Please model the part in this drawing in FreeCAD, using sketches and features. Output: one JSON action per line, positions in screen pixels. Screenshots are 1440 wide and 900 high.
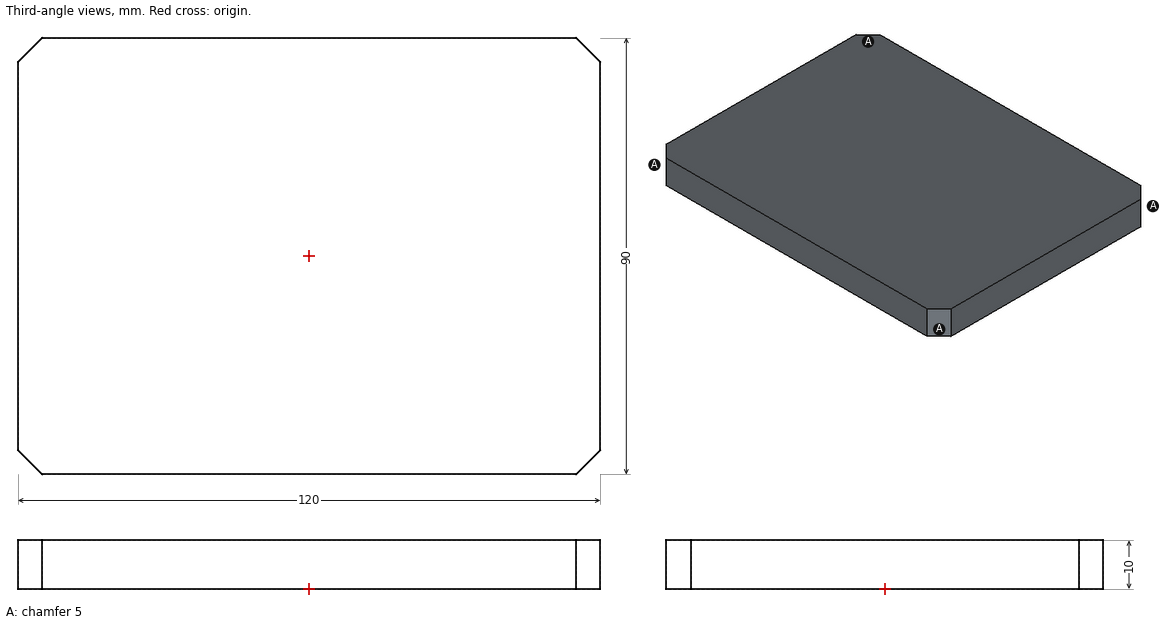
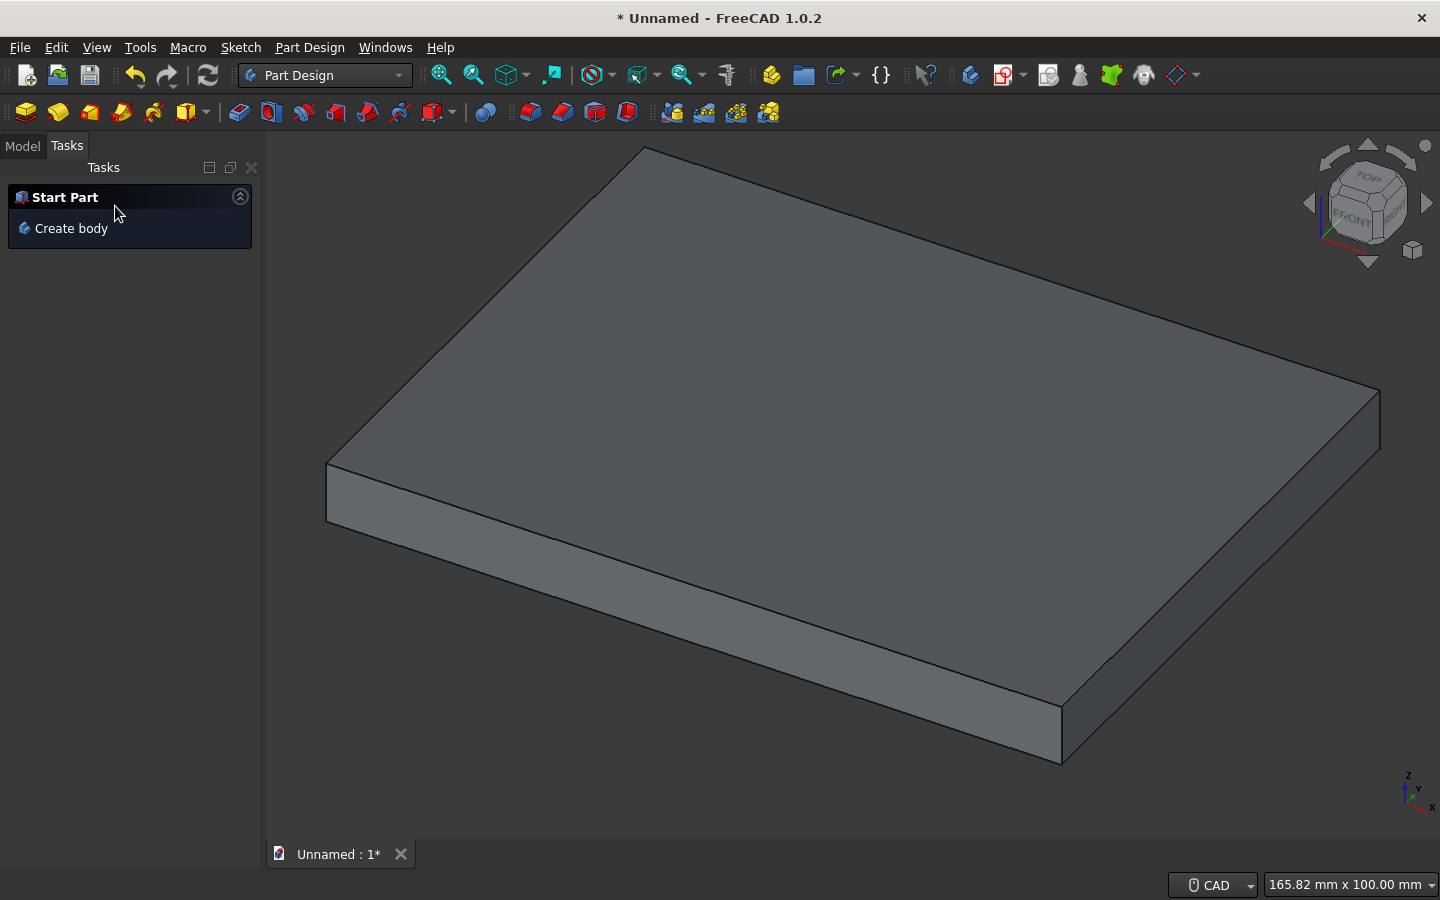
{"action": "left_click", "coordinate": [1062, 735]}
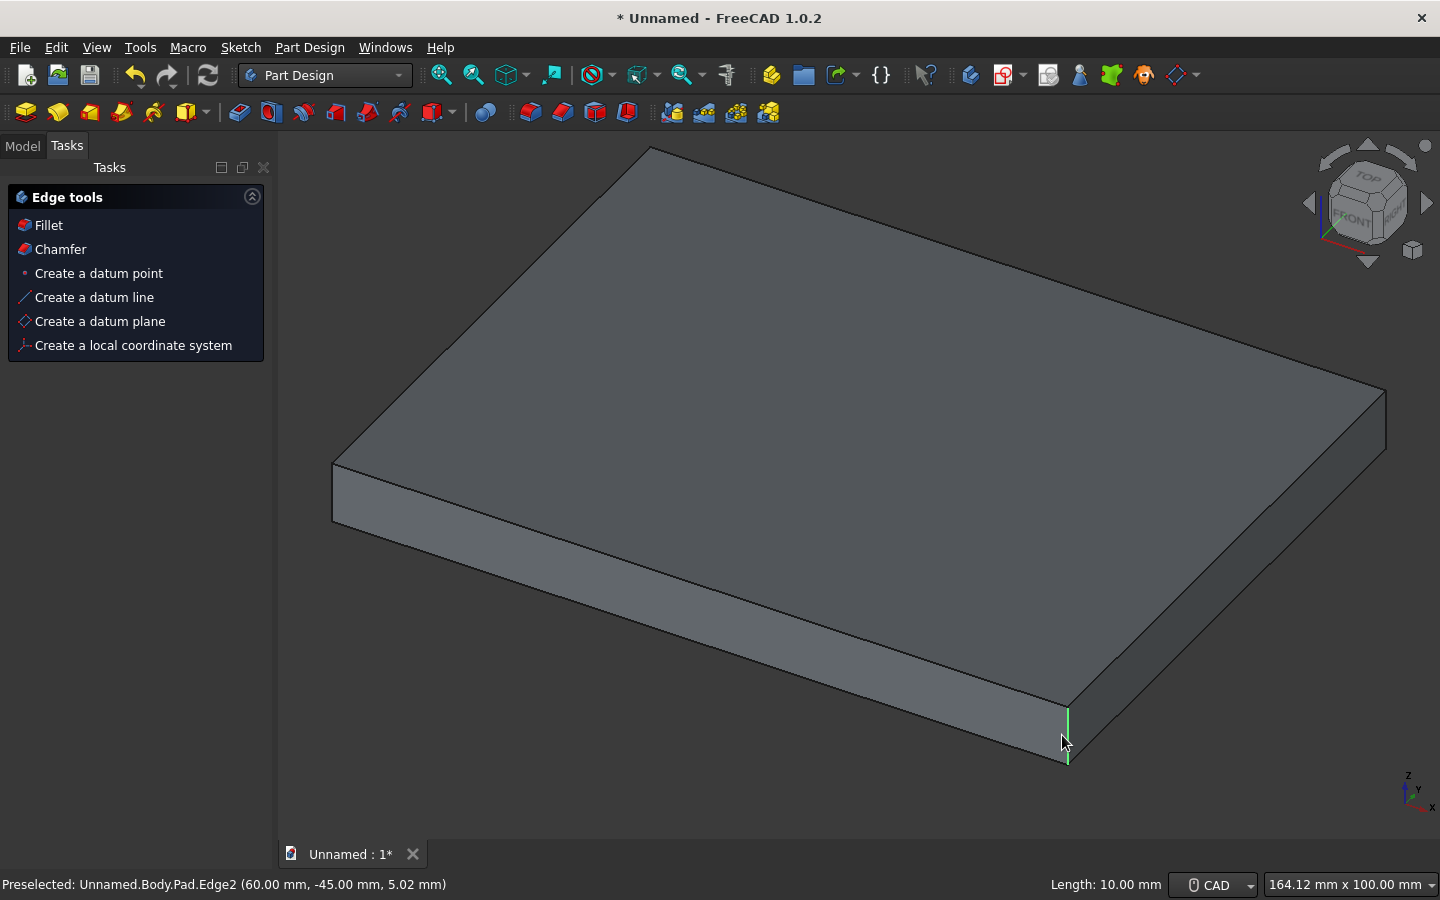
{"action": "key", "text": "0"}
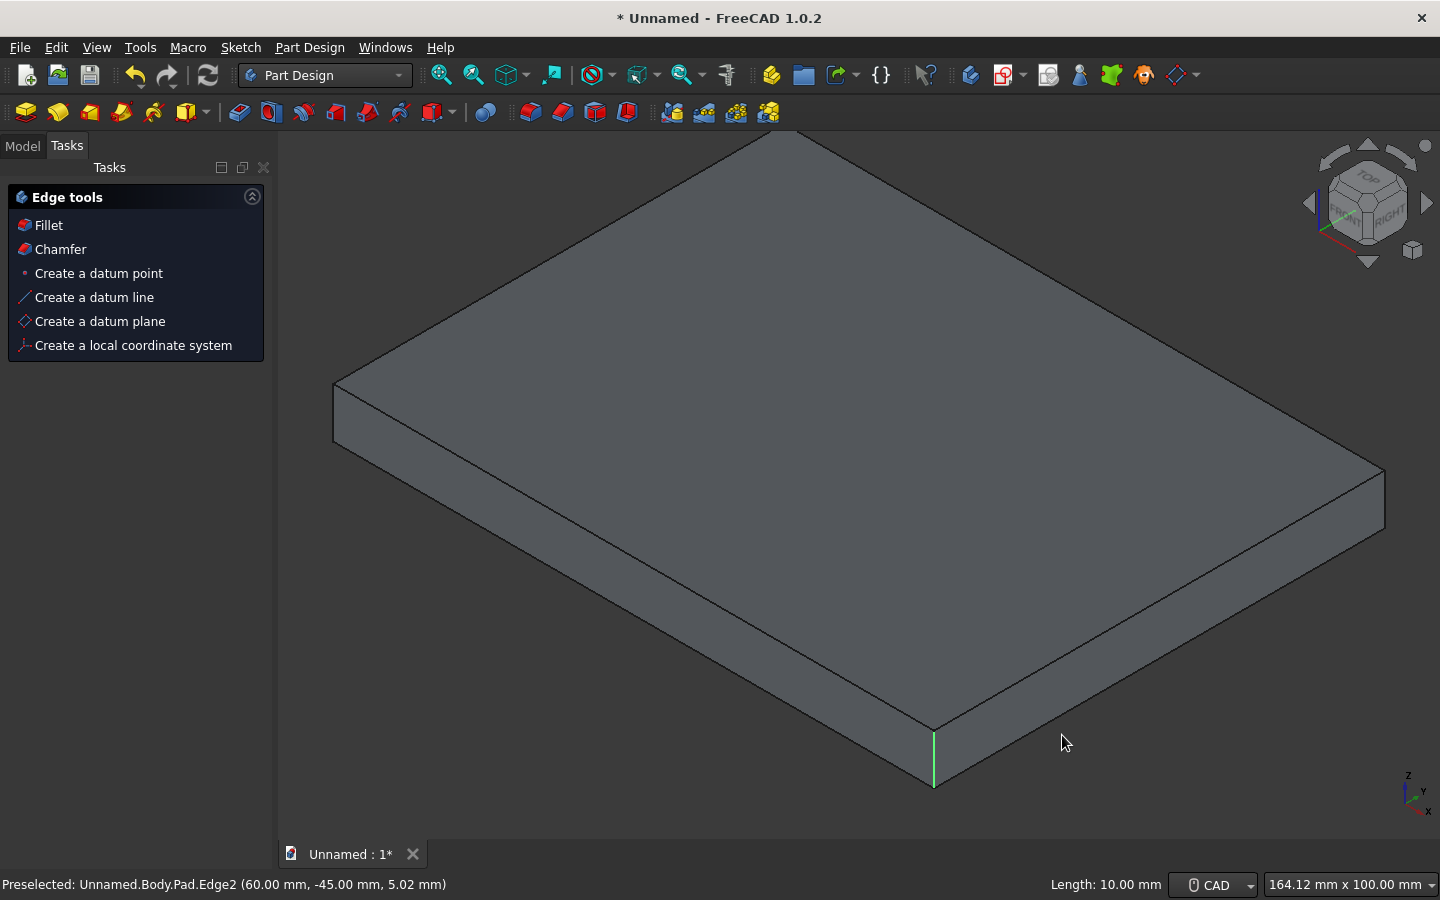
{"action": "left_click", "coordinate": [442, 76]}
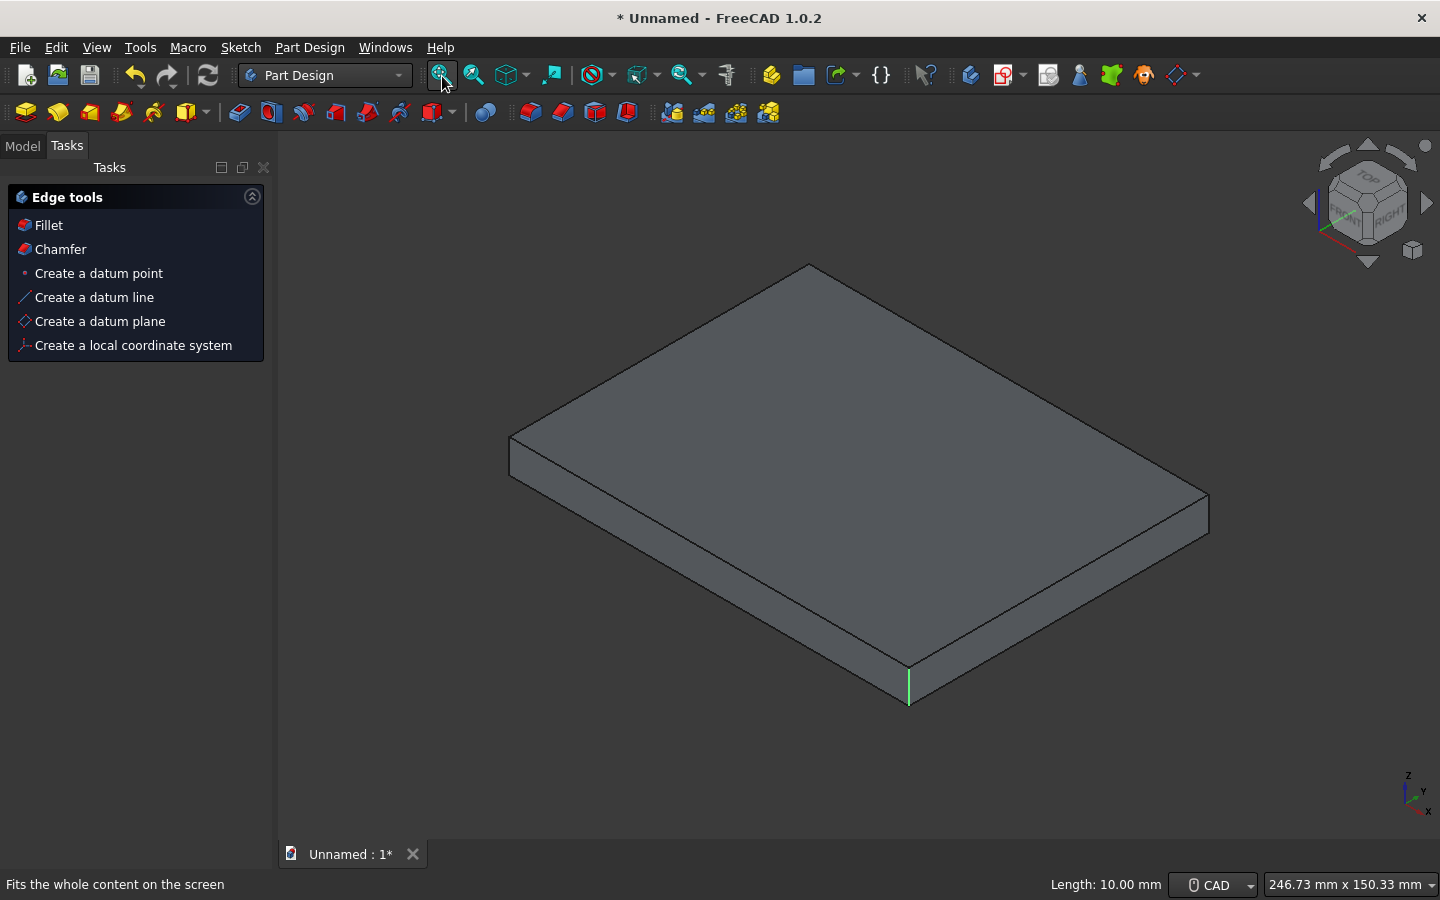
{"action": "key", "text": "2"}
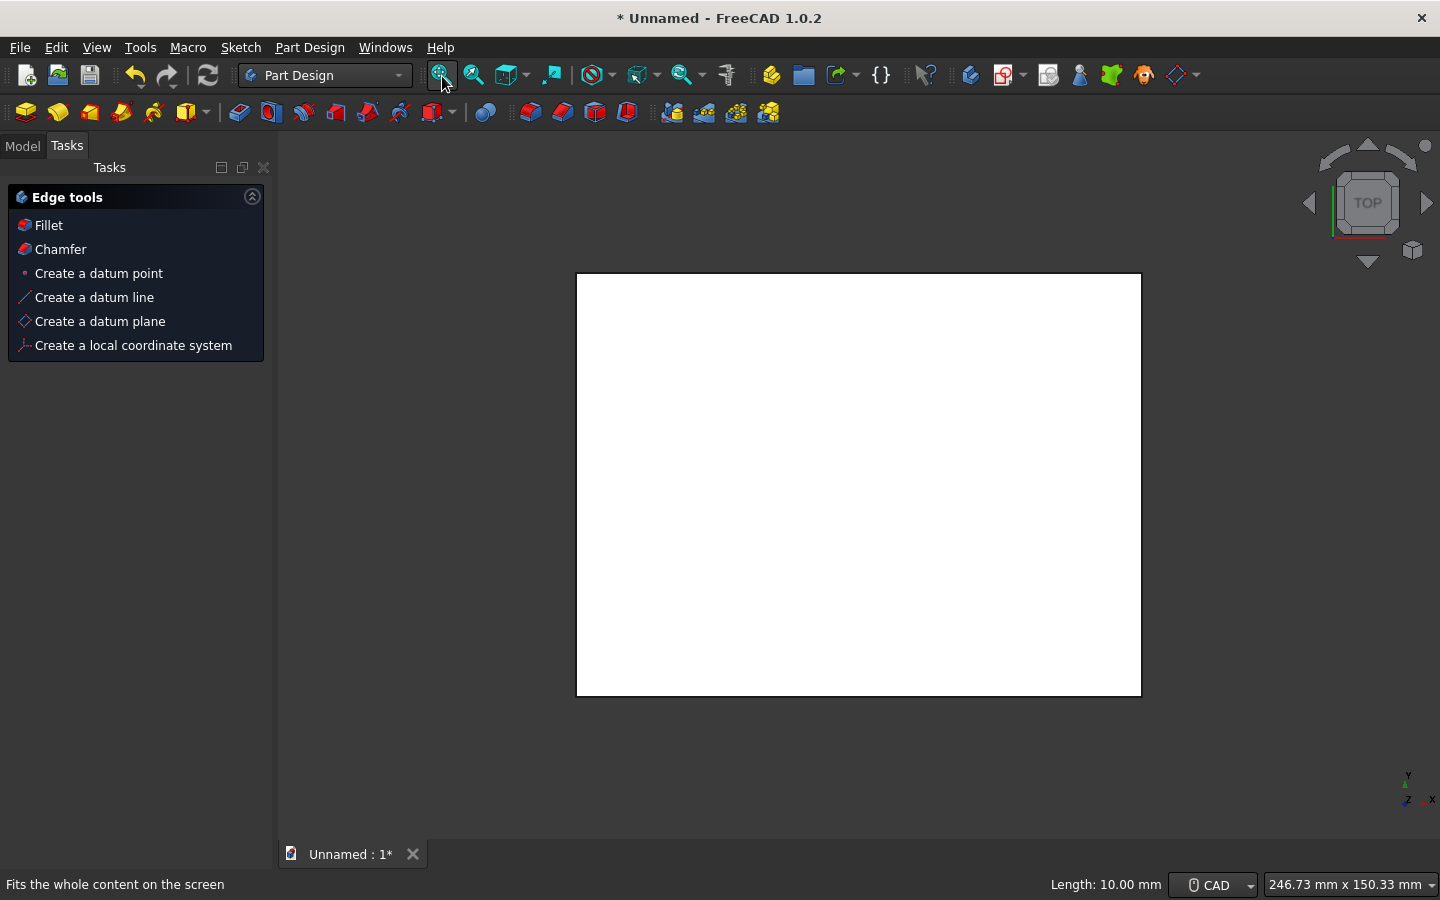
{"action": "key", "text": "1"}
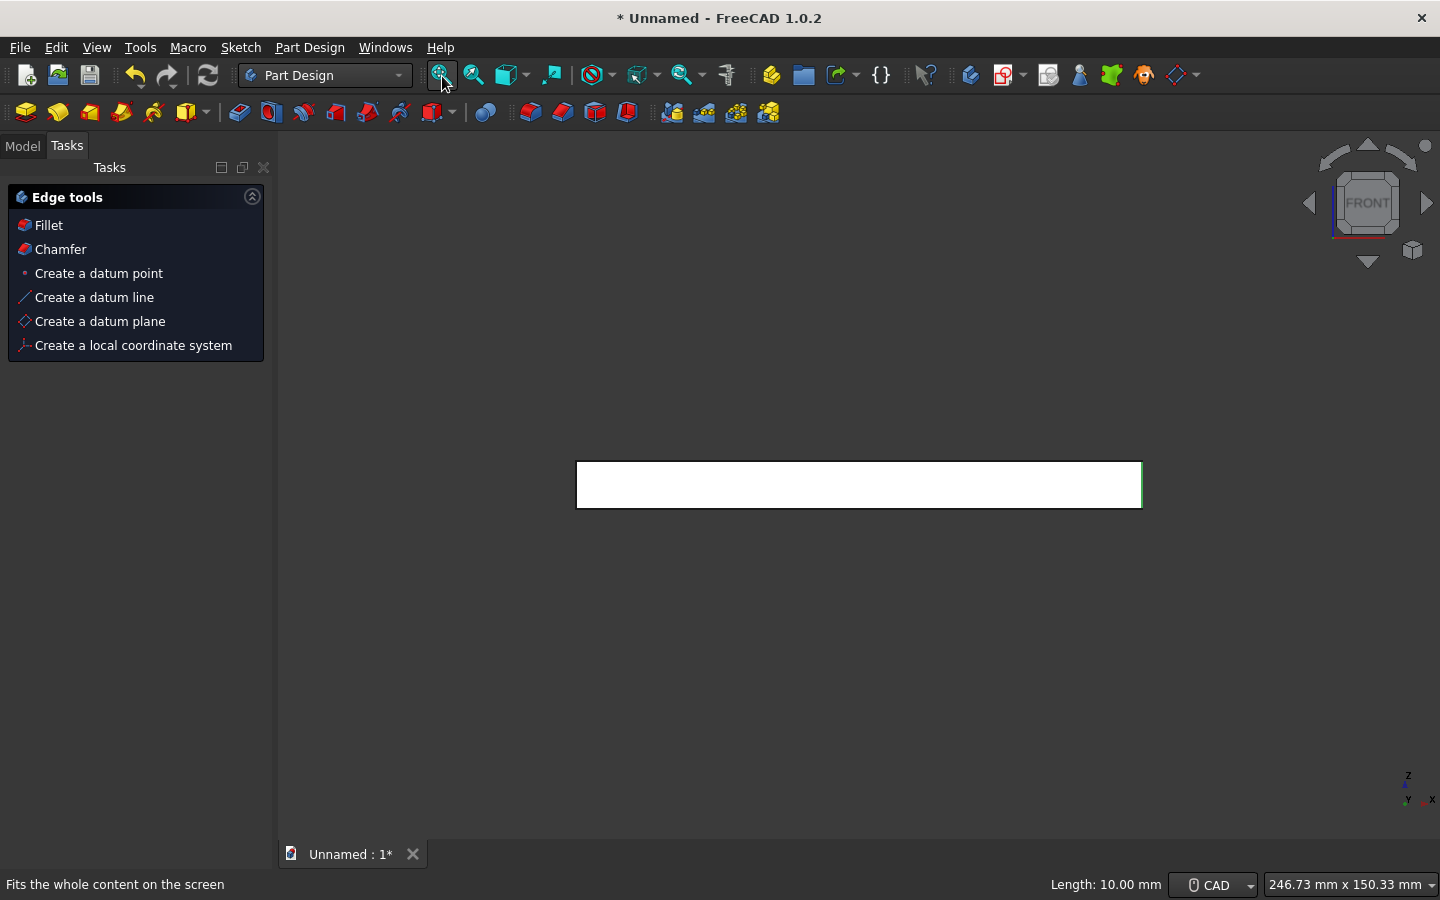
{"action": "left_click", "coordinate": [576, 484], "text": "ctrl"}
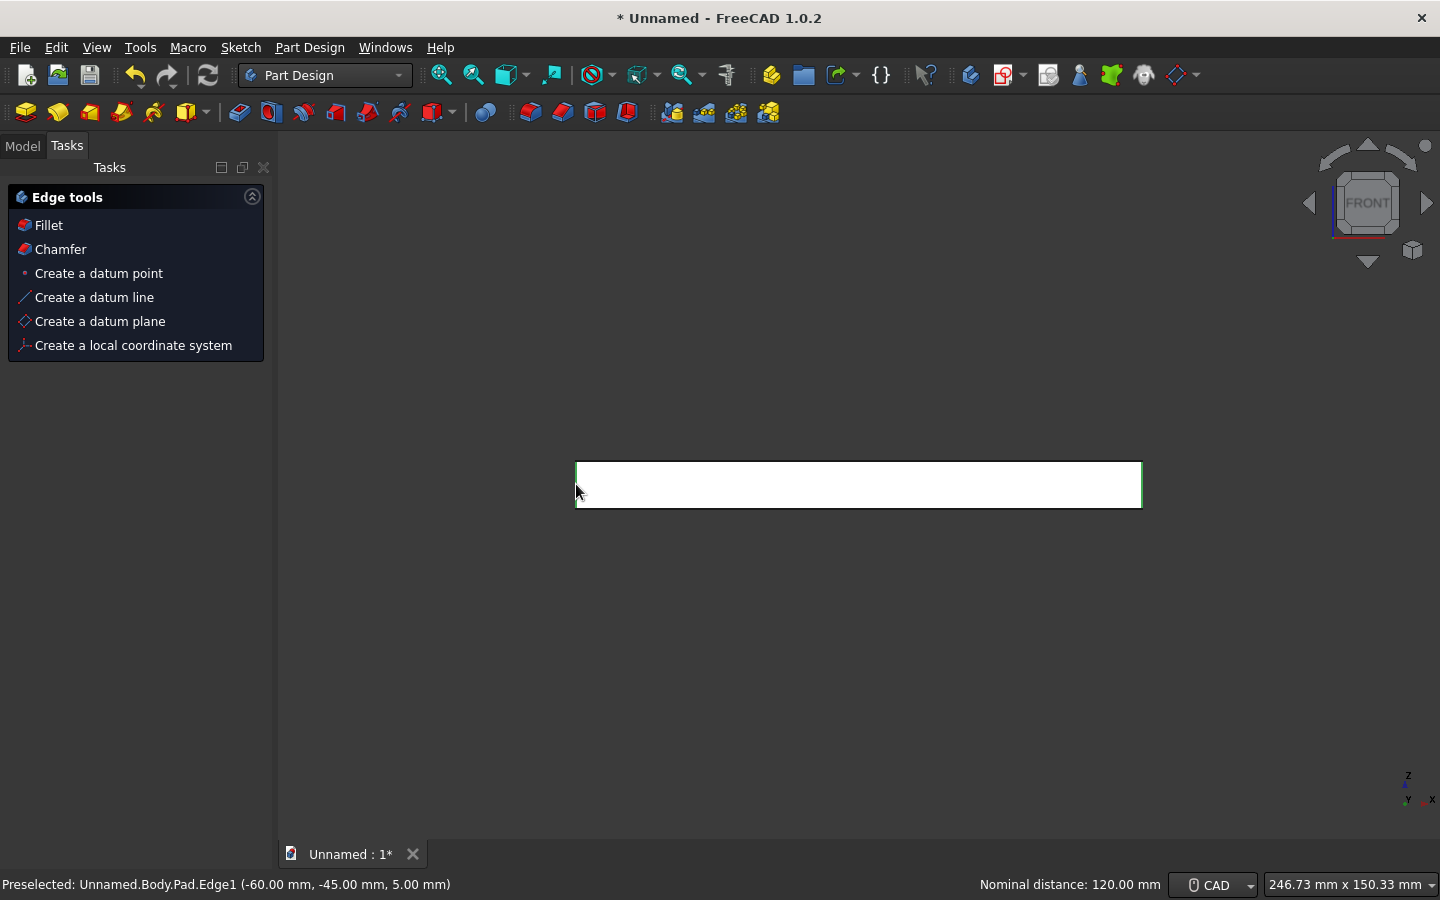
{"action": "key", "text": "3"}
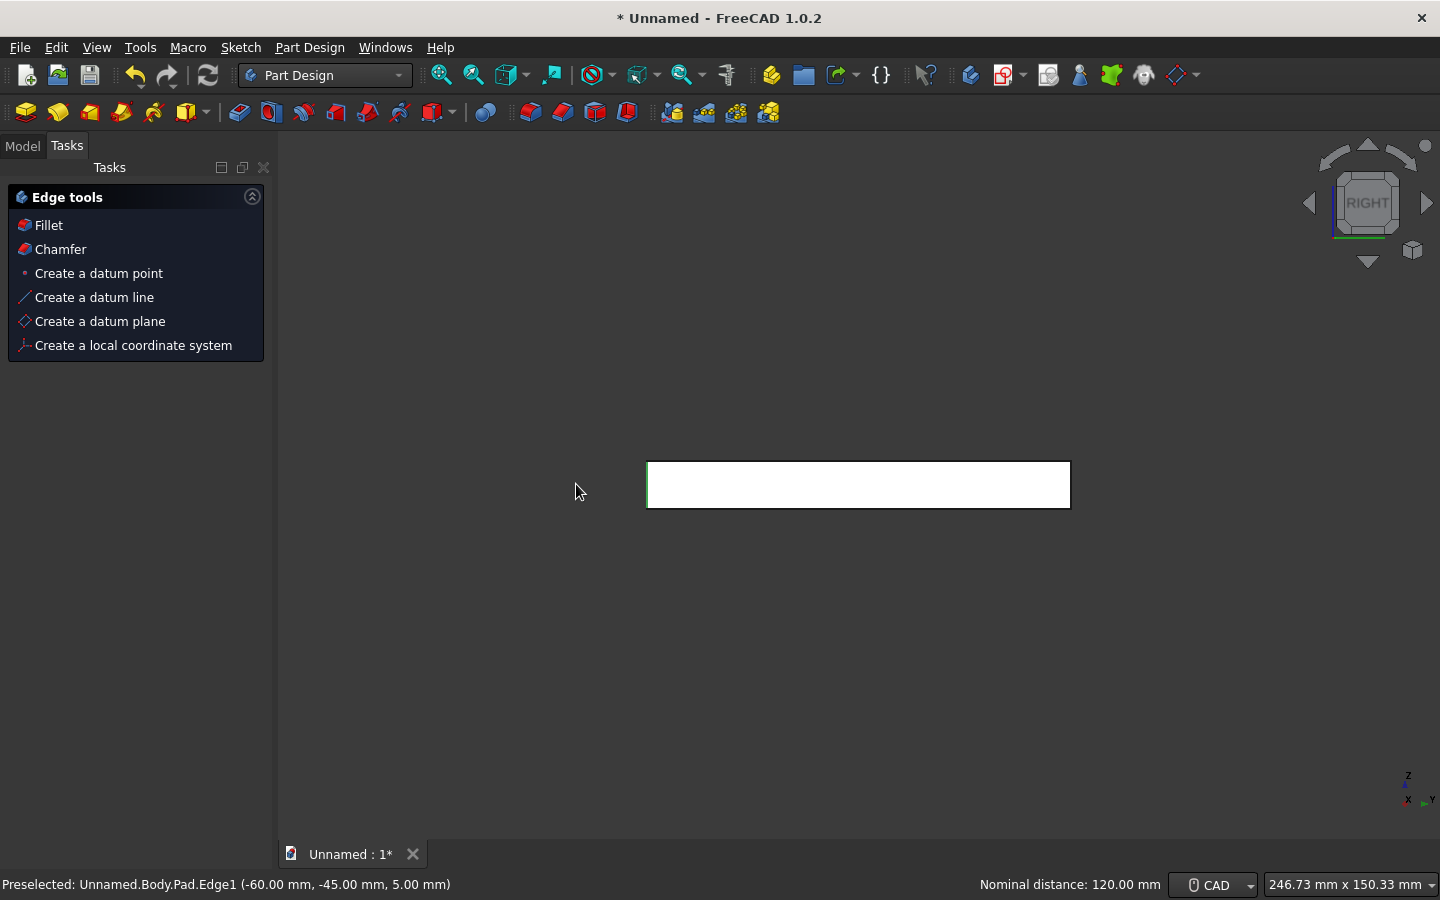
{"action": "left_click", "coordinate": [442, 76]}